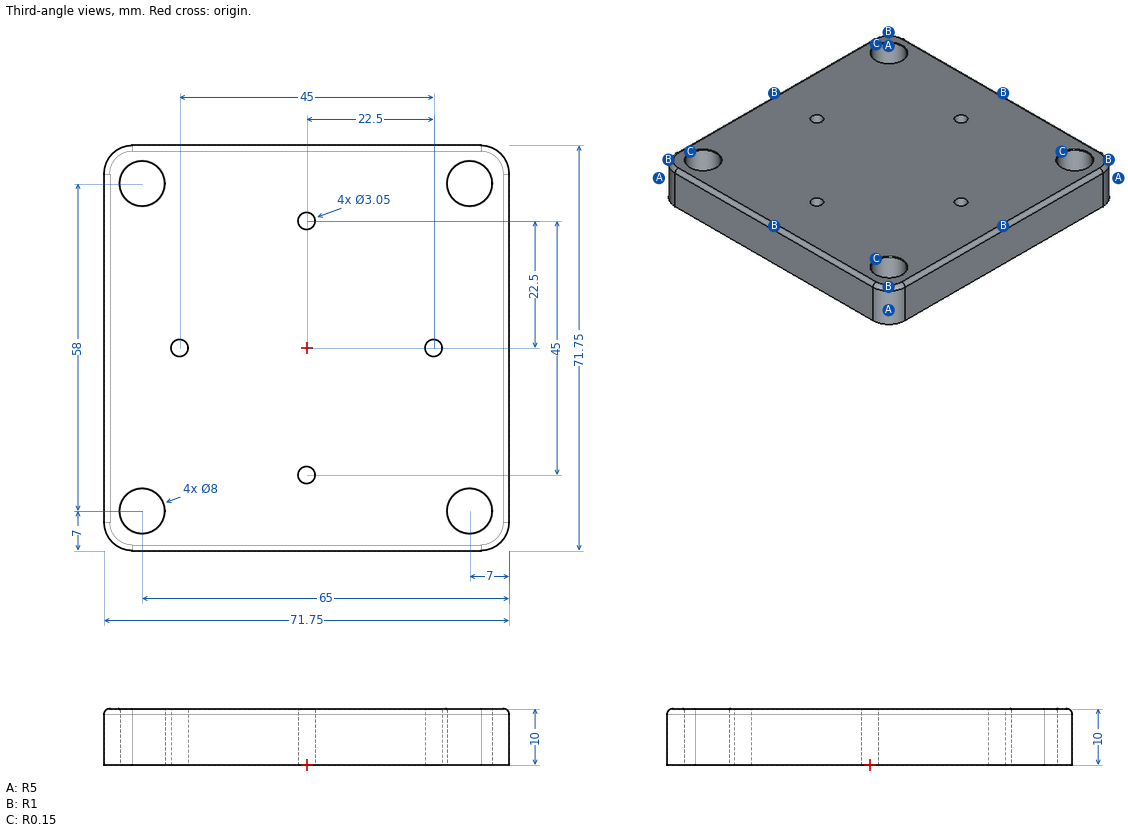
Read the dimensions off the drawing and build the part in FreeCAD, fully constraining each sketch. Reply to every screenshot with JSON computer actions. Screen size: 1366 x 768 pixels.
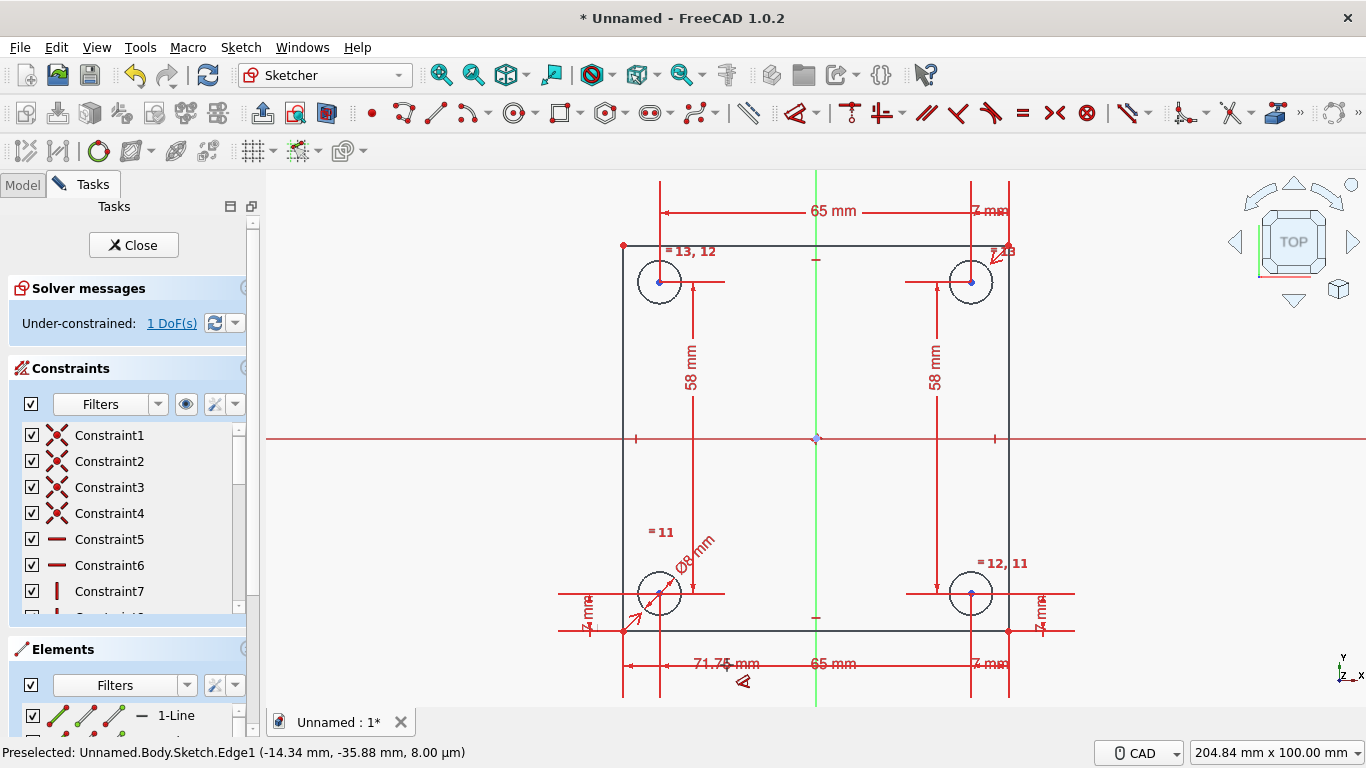
{"action": "left_click", "coordinate": [1009, 516]}
{"action": "left_click", "coordinate": [1043, 350]}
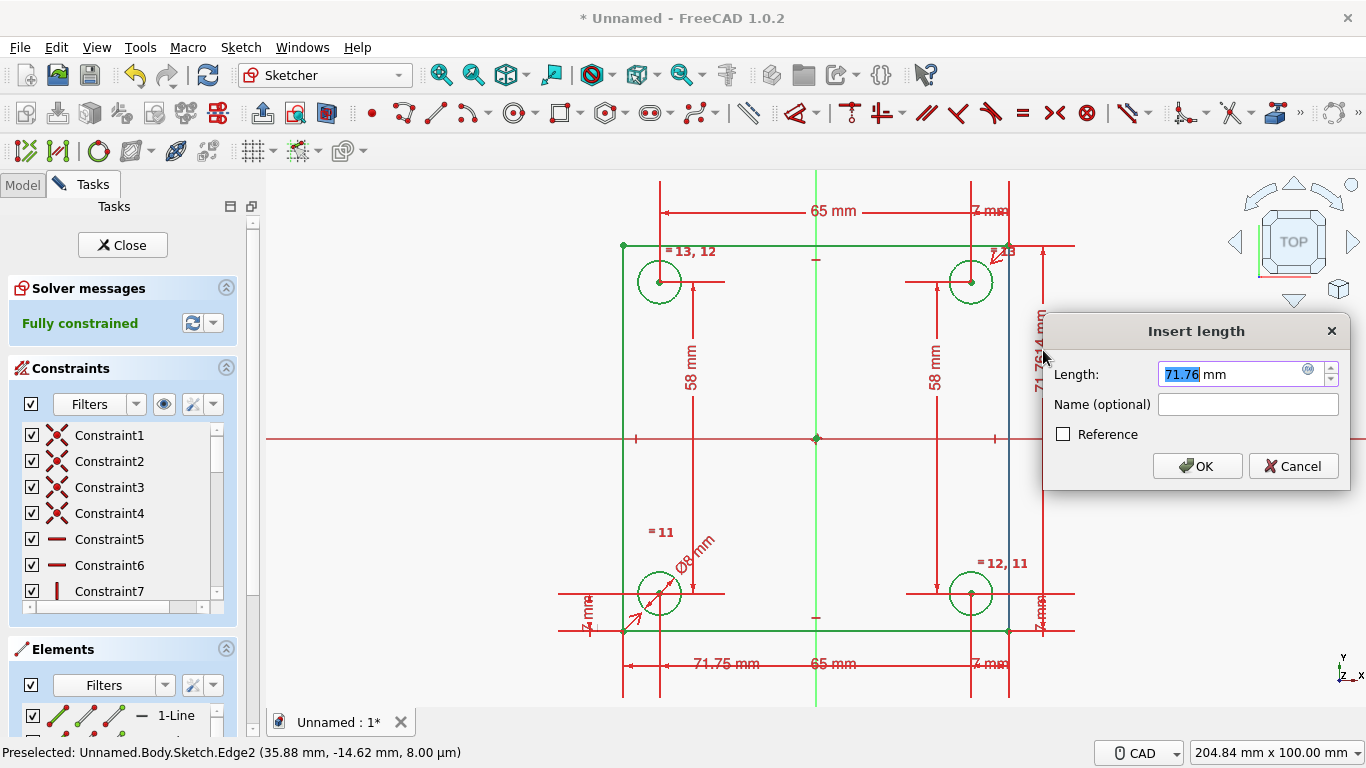
{"action": "type", "text": "71.75"}
{"action": "key", "text": "Return"}
{"action": "key", "text": "Escape"}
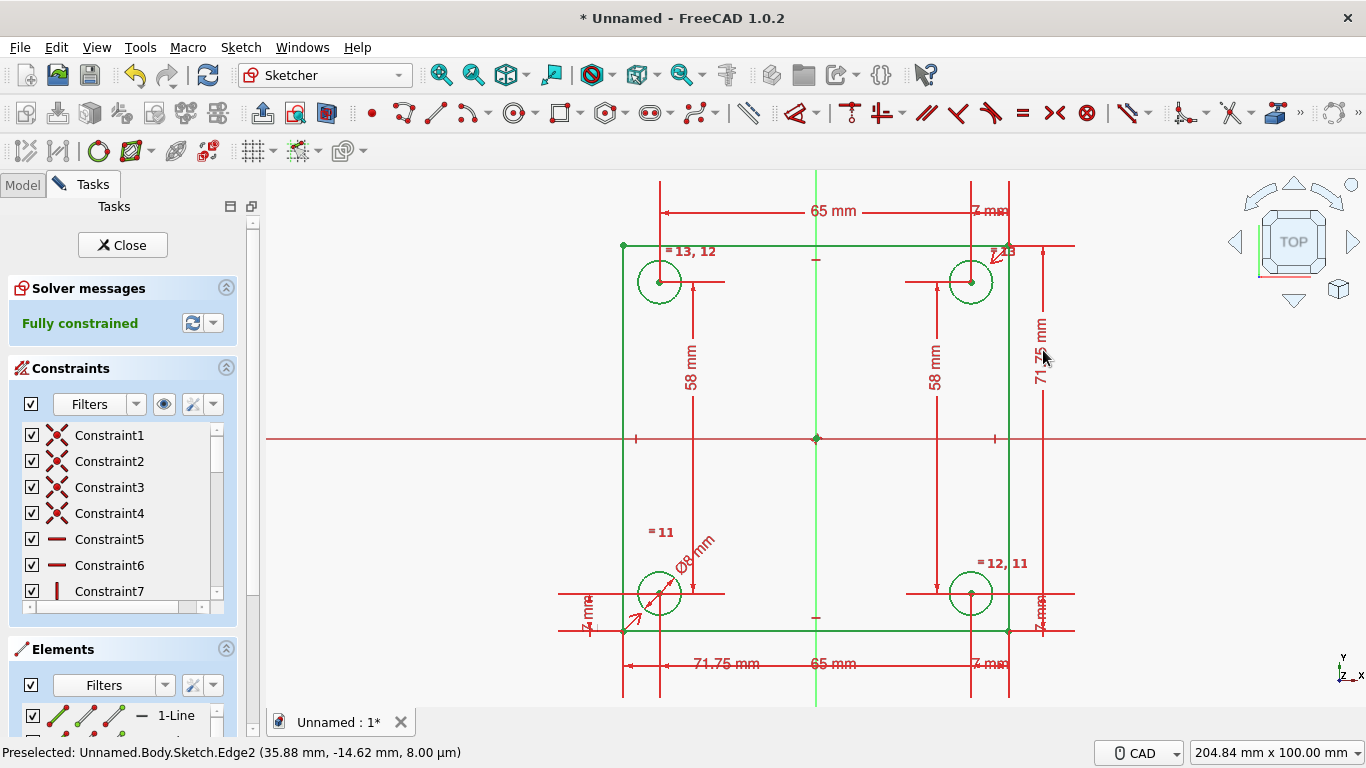
{"action": "left_click", "coordinate": [123, 245]}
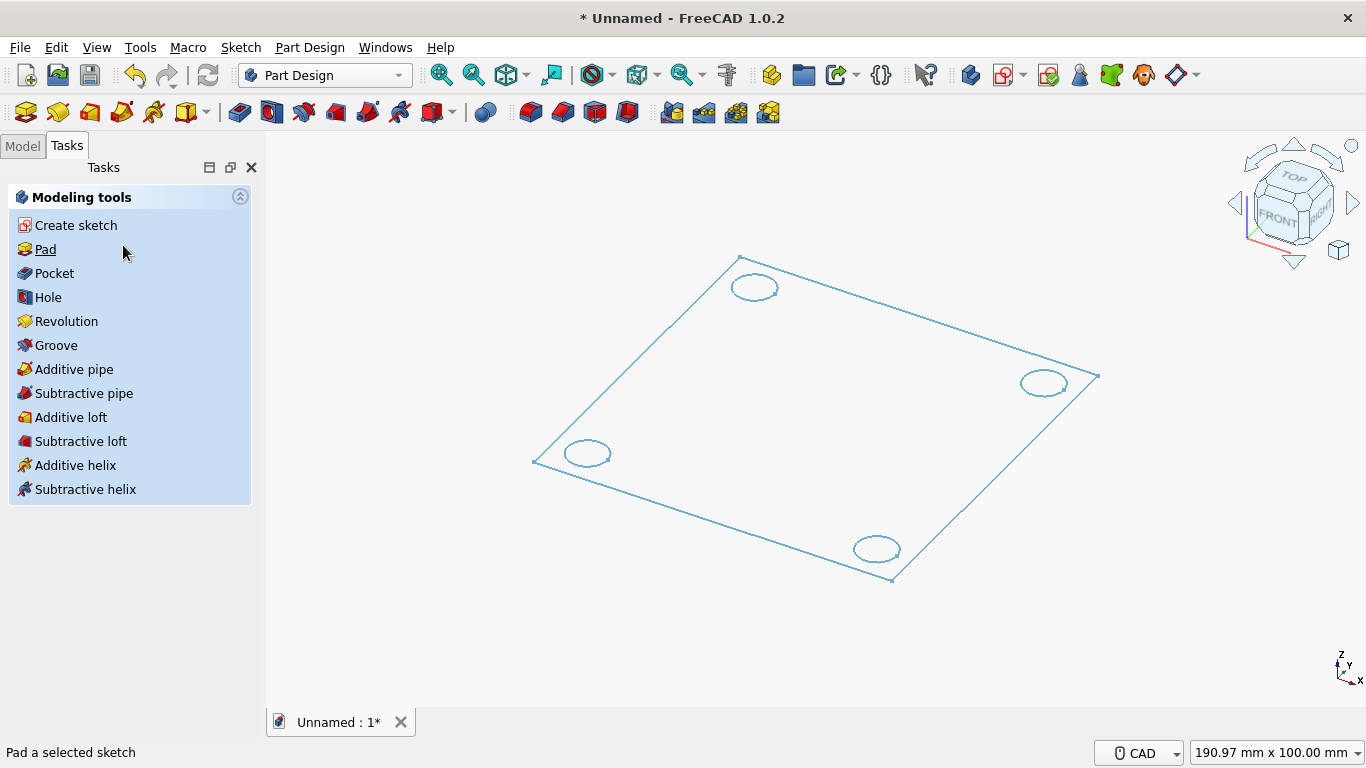
{"action": "left_click", "coordinate": [26, 112]}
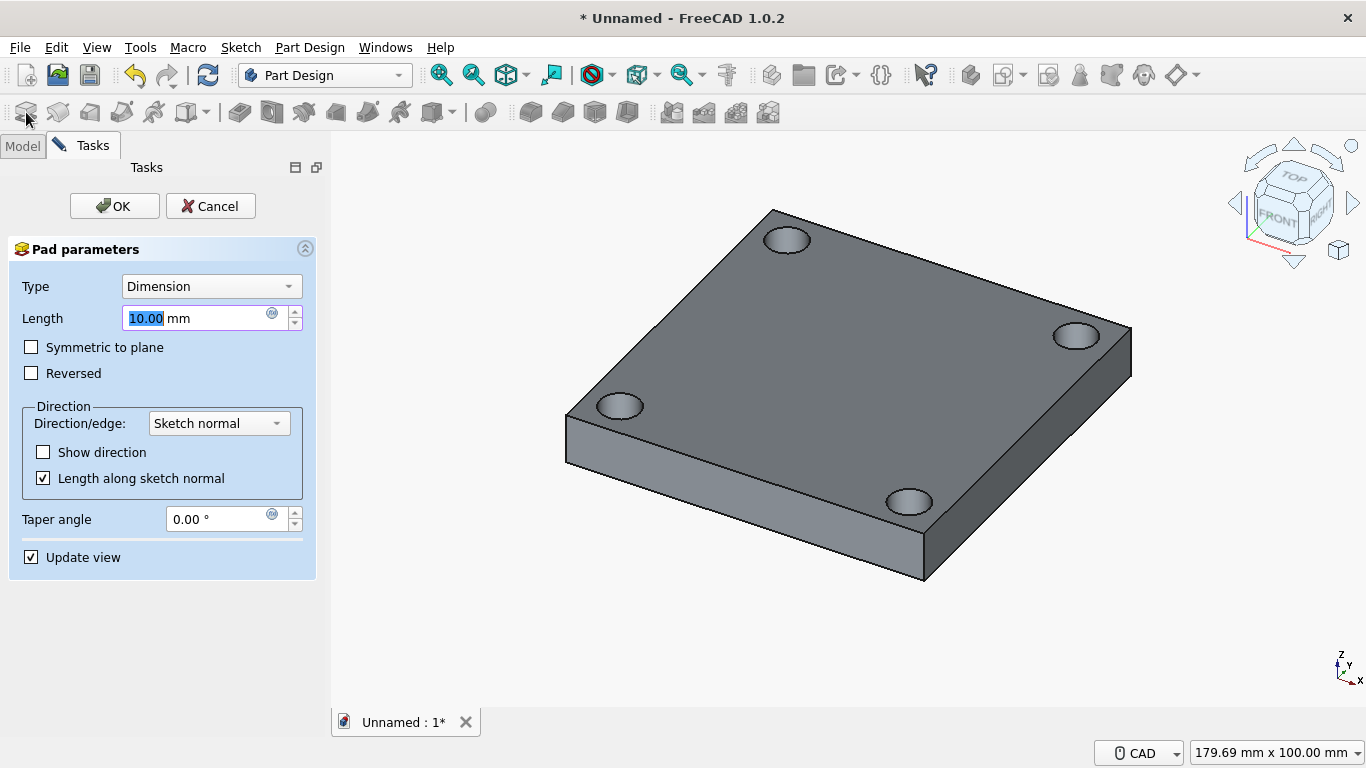
{"action": "type", "text": "10"}
{"action": "key", "text": "Tab"}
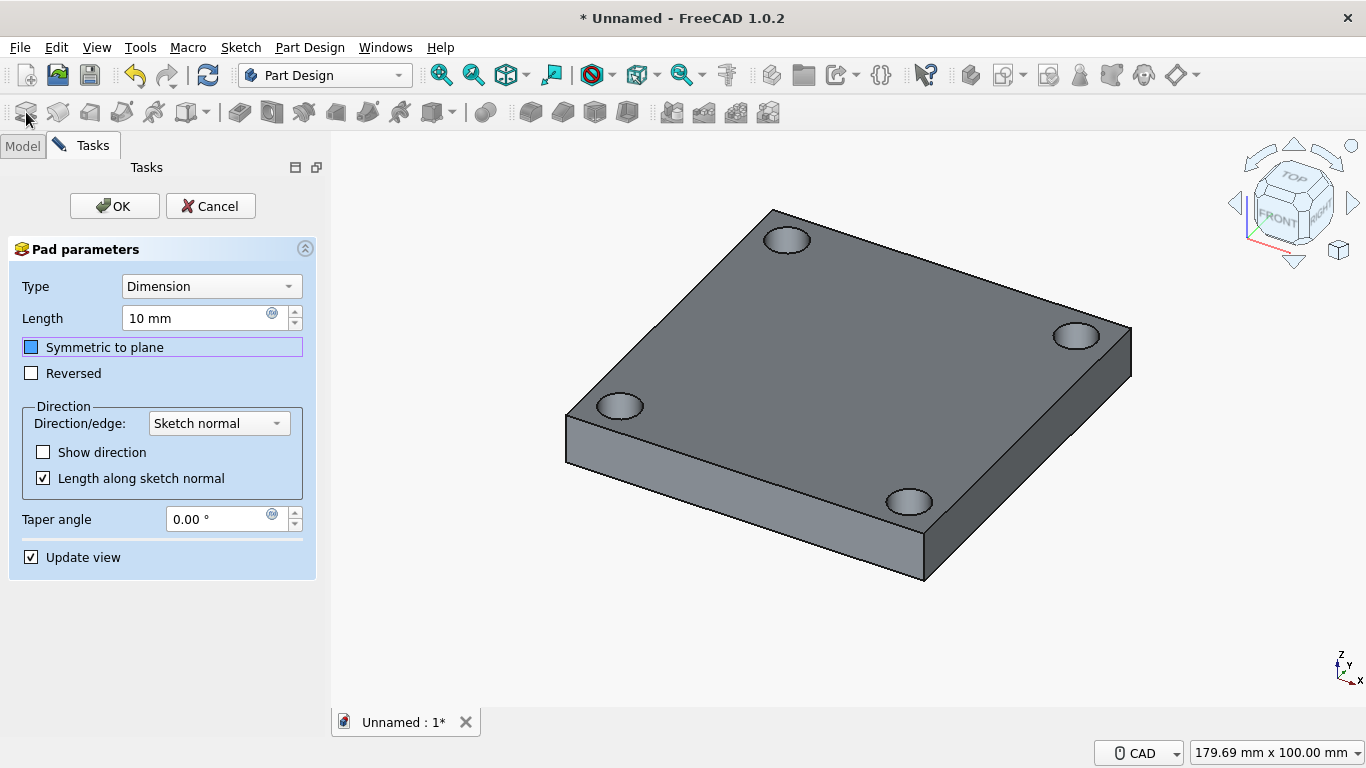
{"action": "left_click", "coordinate": [115, 206]}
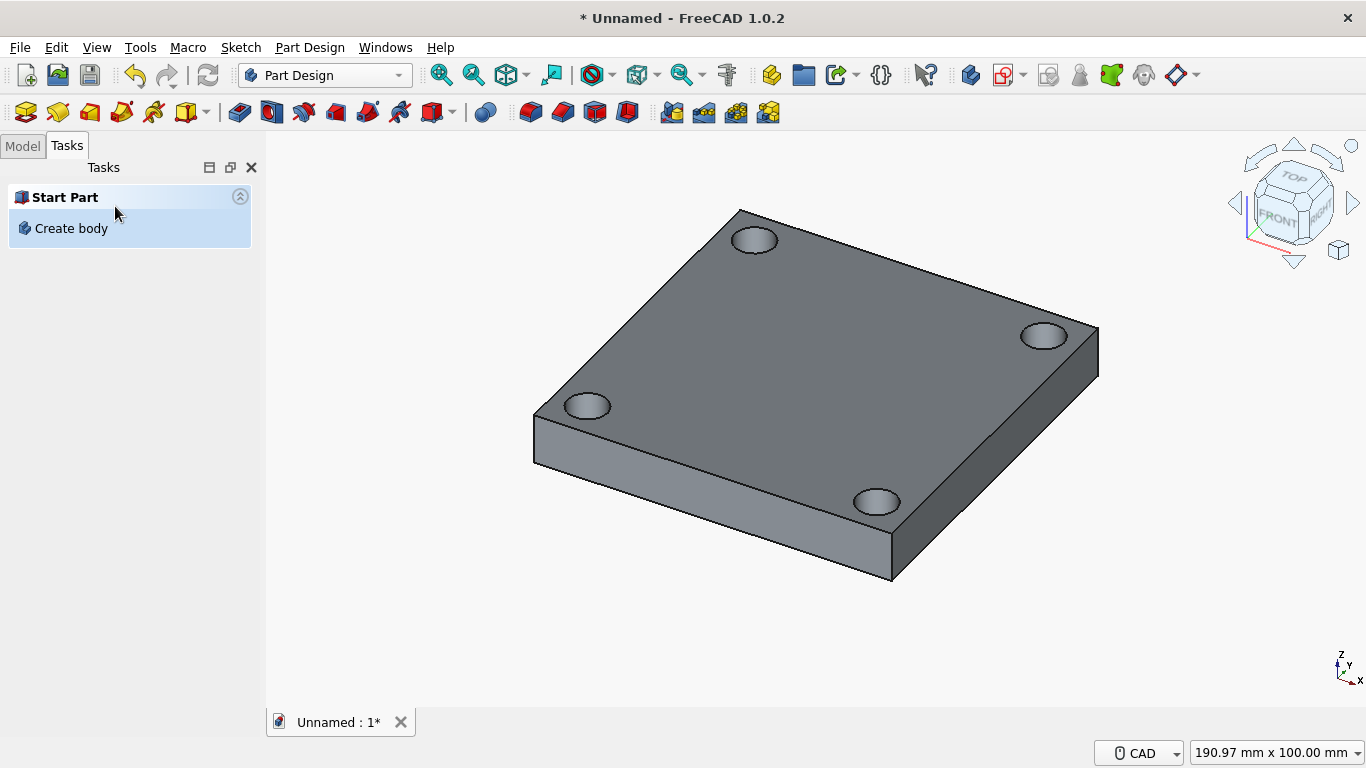
{"action": "left_click", "coordinate": [892, 556]}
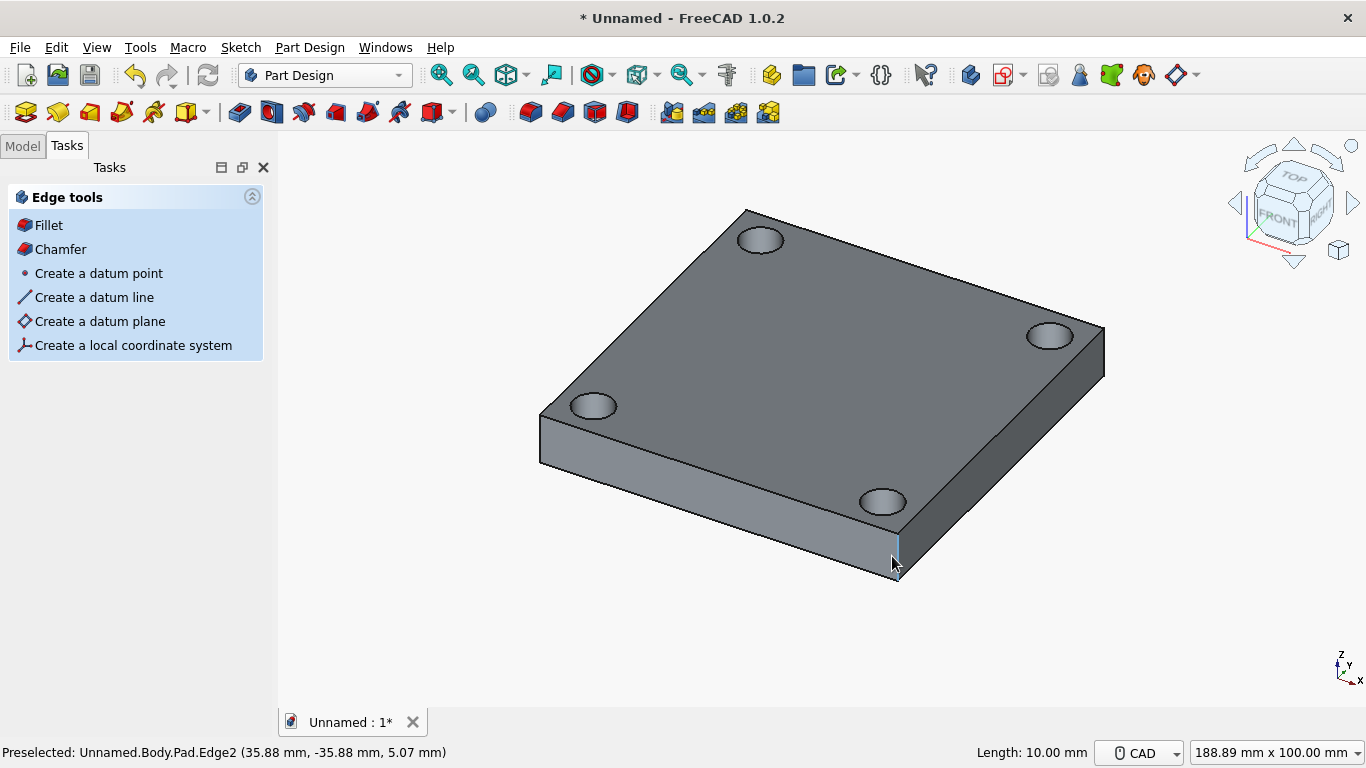
{"action": "key", "text": "0"}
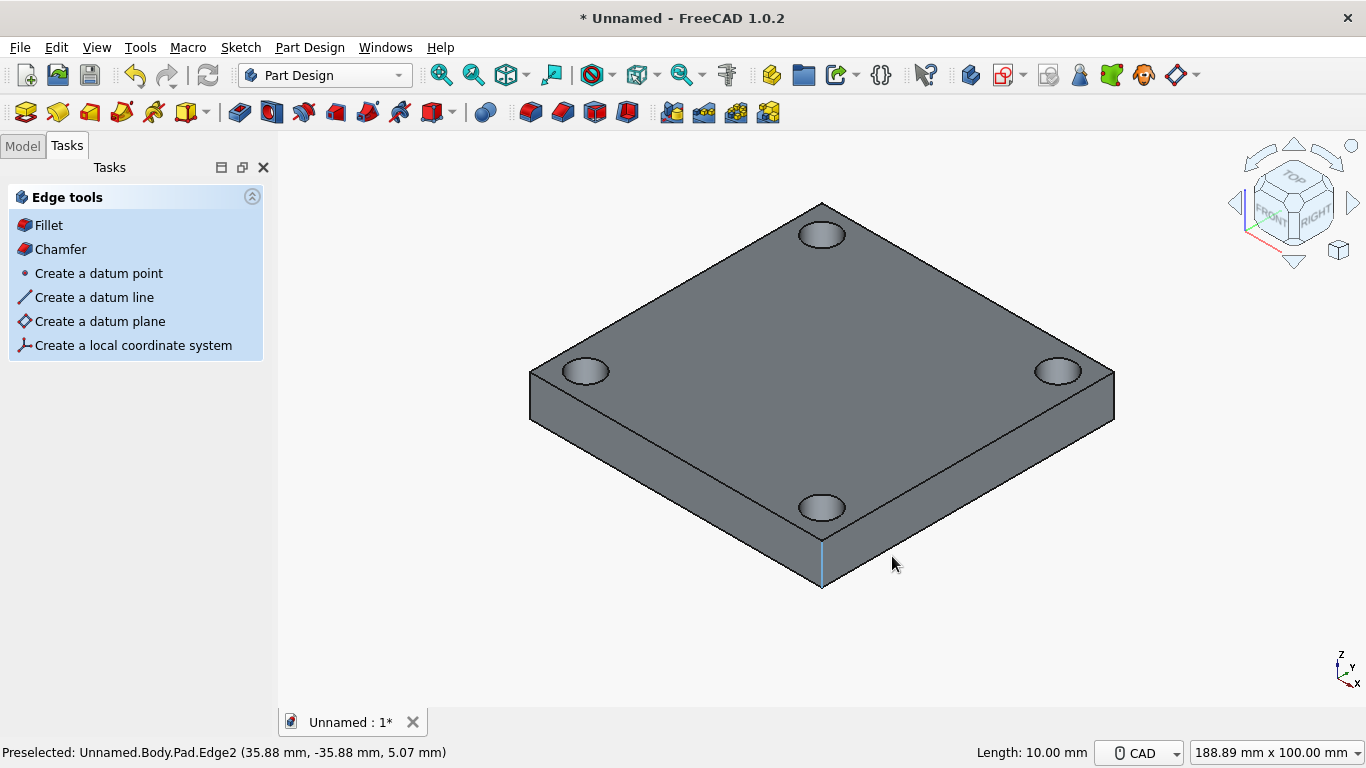
{"action": "key", "text": "2"}